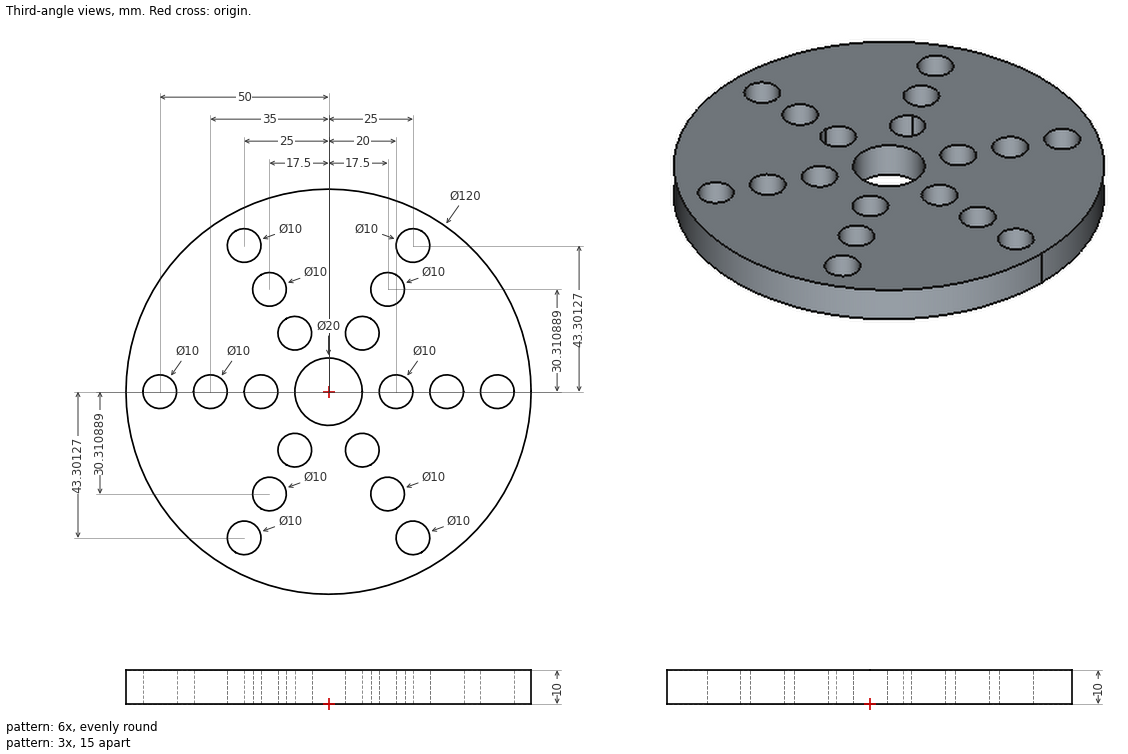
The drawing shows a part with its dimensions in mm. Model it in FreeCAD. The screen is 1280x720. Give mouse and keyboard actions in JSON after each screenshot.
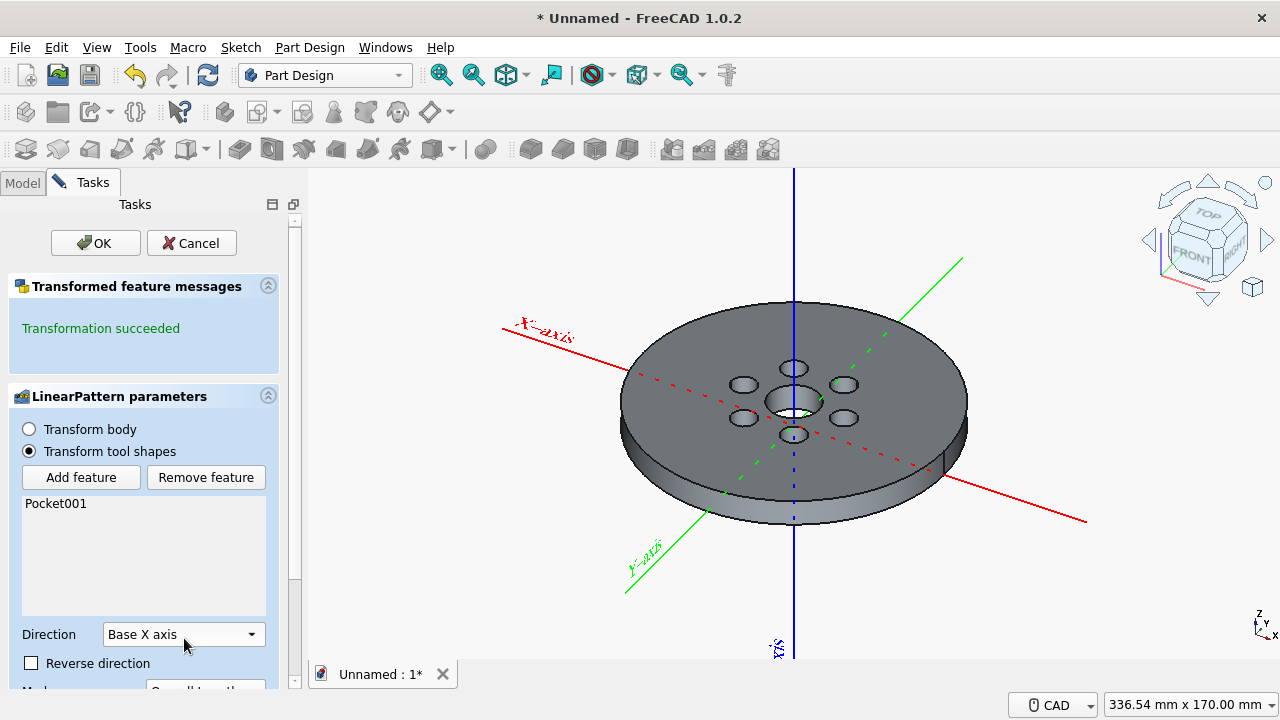
{"action": "scroll", "coordinate": [295, 451], "scroll_direction": "down", "scroll_amount": 2}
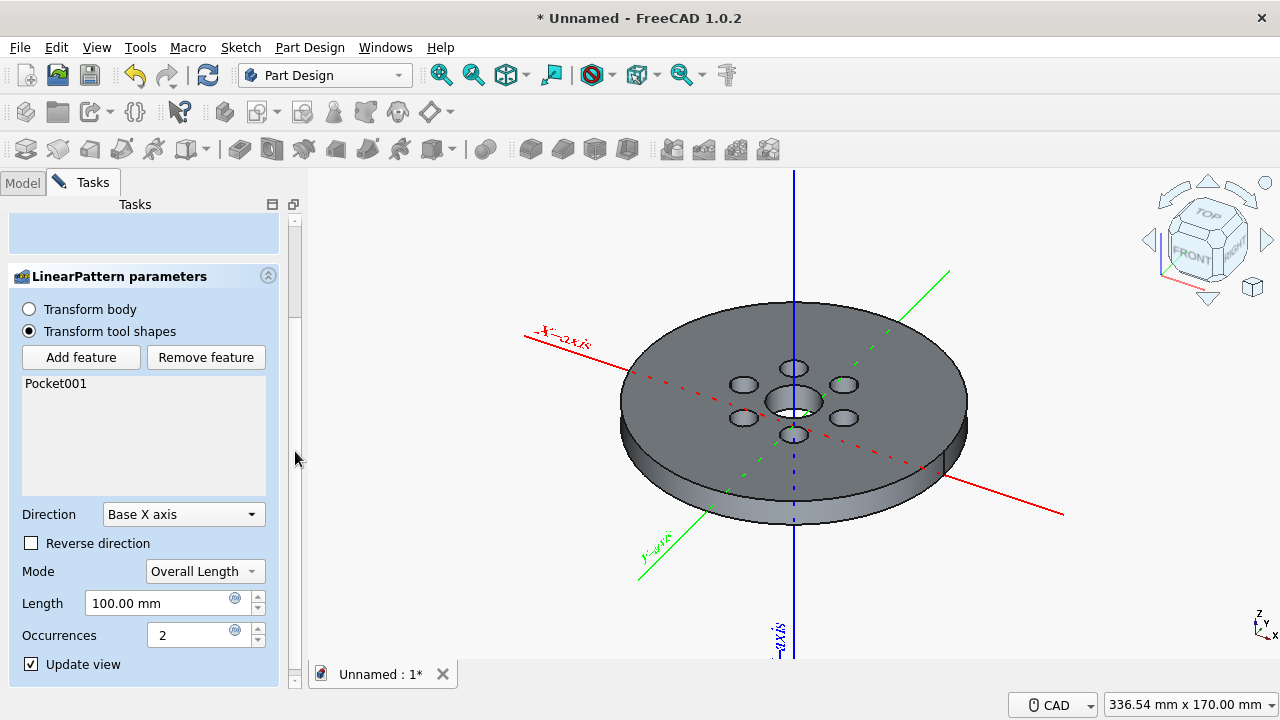
{"action": "left_click", "coordinate": [206, 572]}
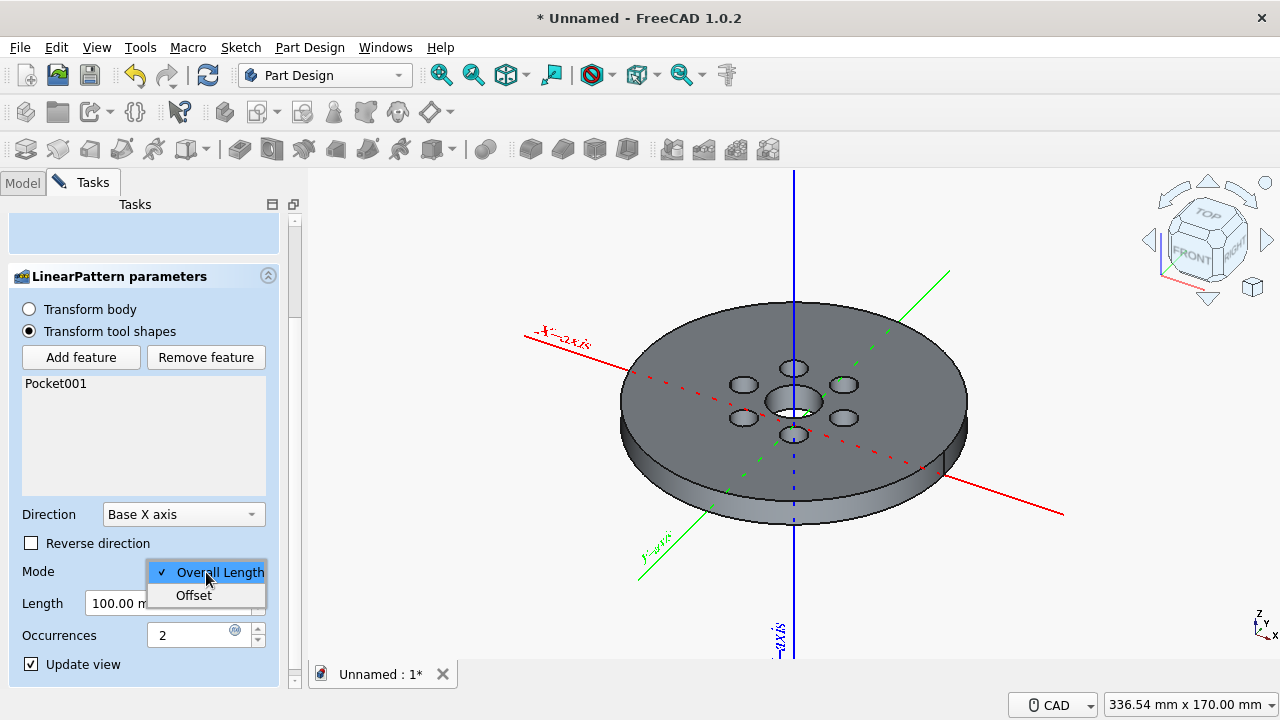
{"action": "left_click", "coordinate": [206, 596]}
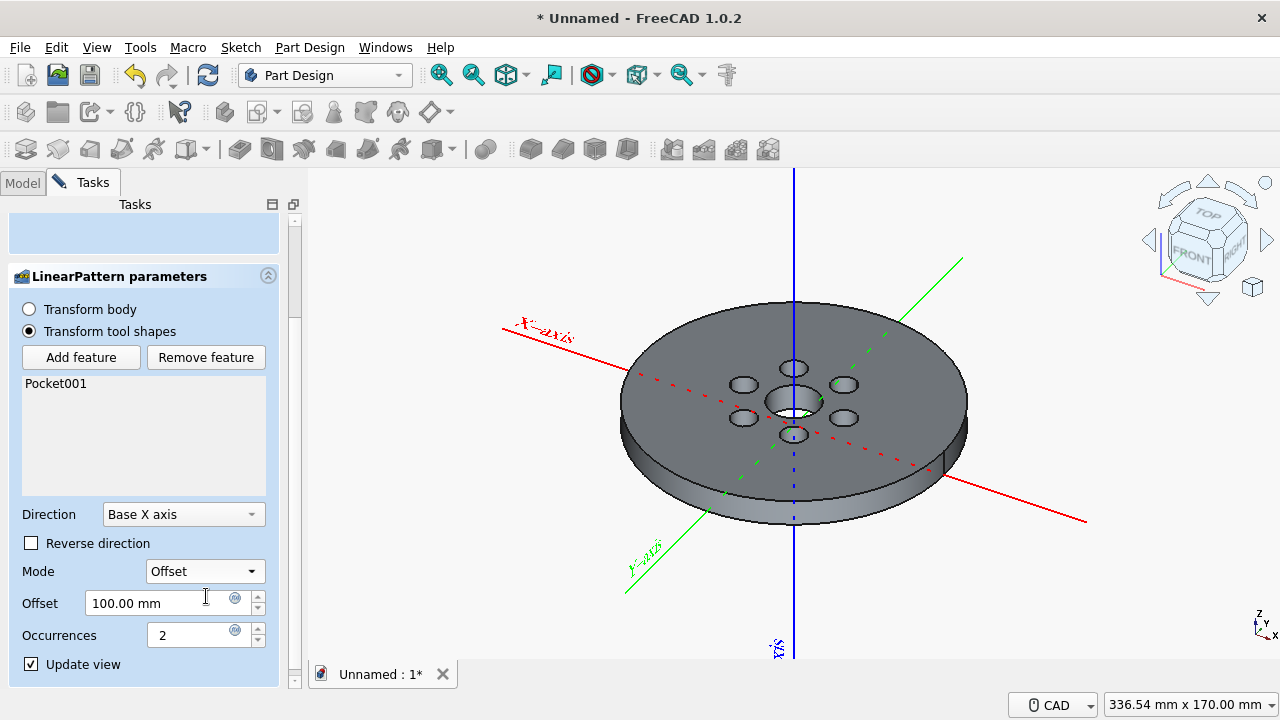
{"action": "triple_click", "coordinate": [168, 603]}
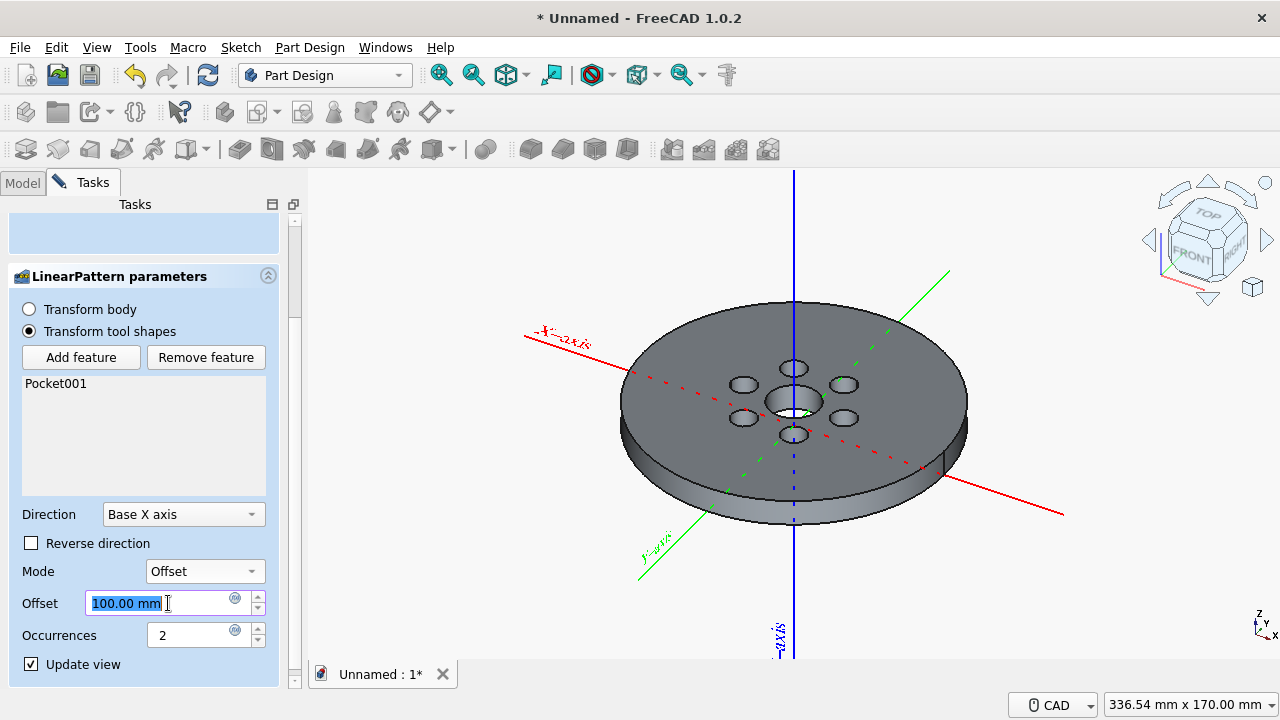
{"action": "type", "text": "15"}
{"action": "key", "text": "Tab"}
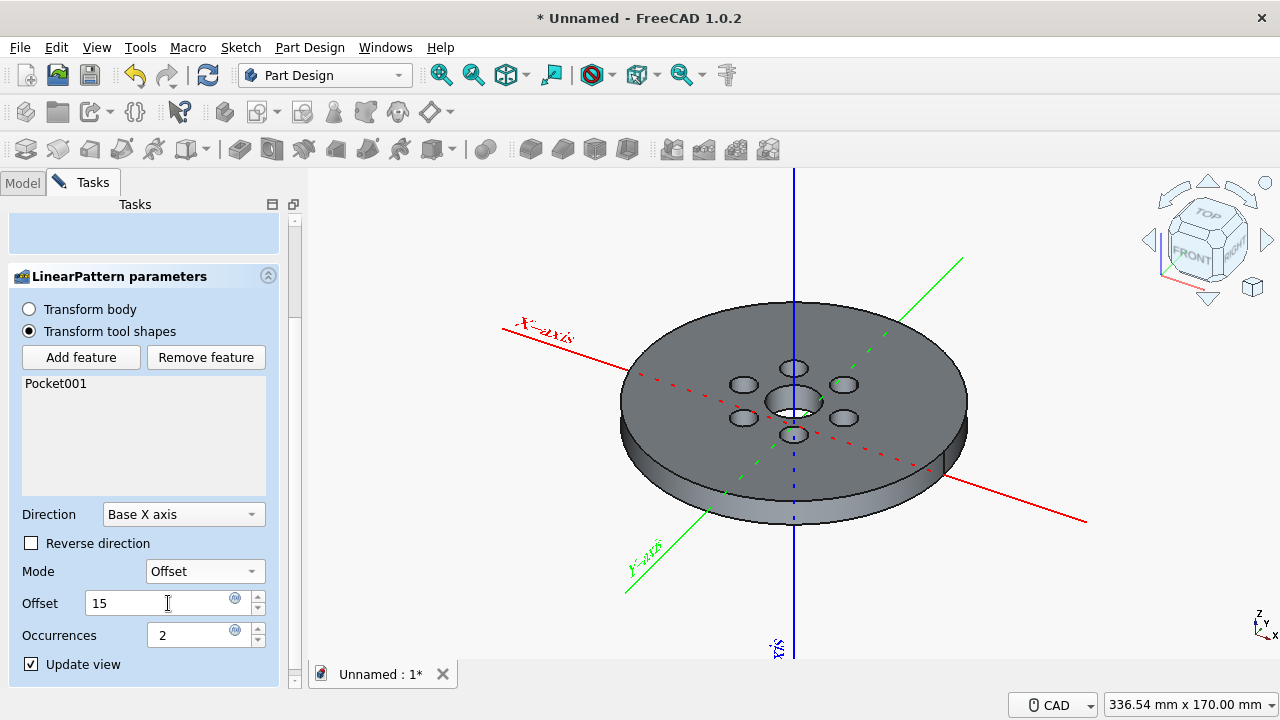
{"action": "triple_click", "coordinate": [198, 635]}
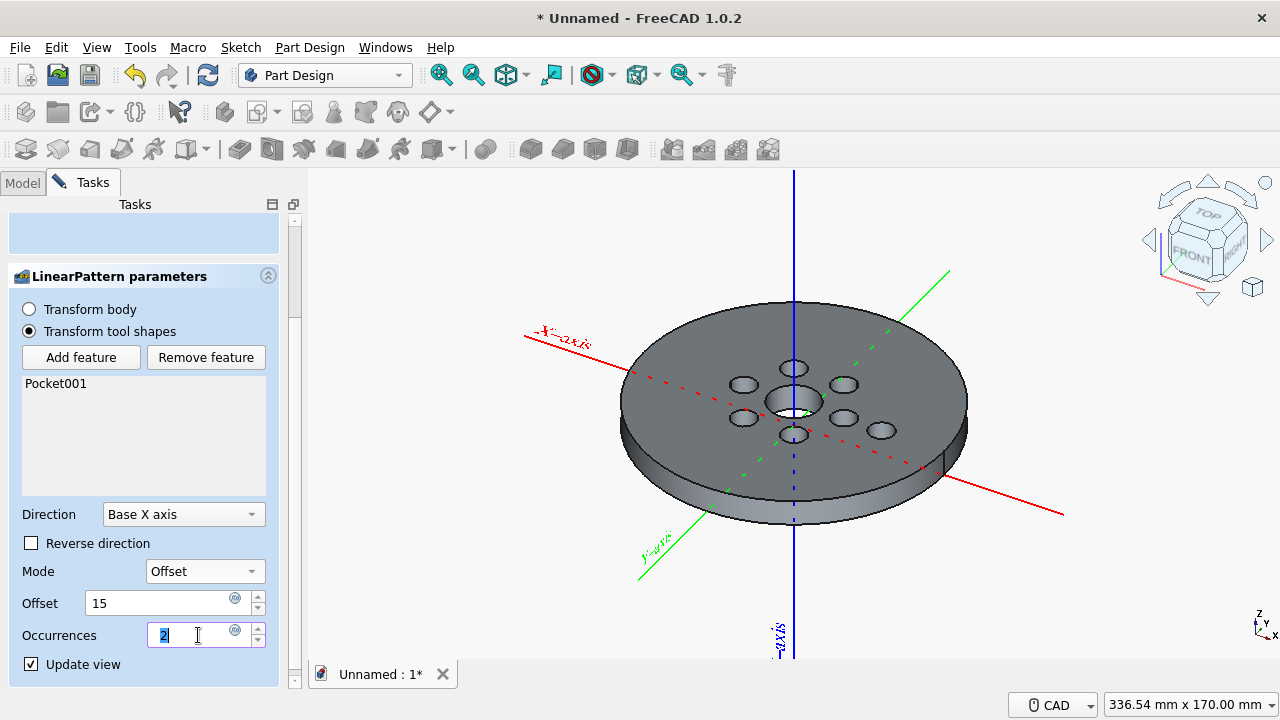
{"action": "type", "text": "3"}
{"action": "key", "text": "Tab"}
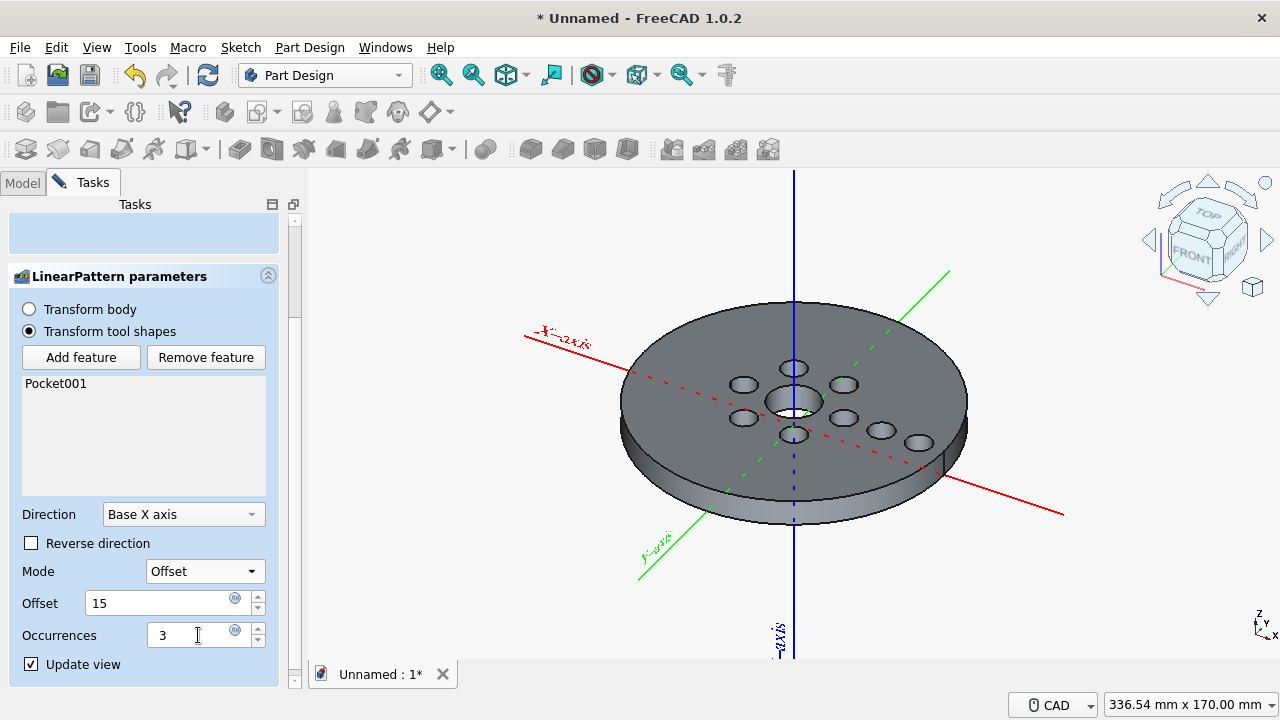
{"action": "scroll", "coordinate": [295, 451], "scroll_direction": "up", "scroll_amount": 3}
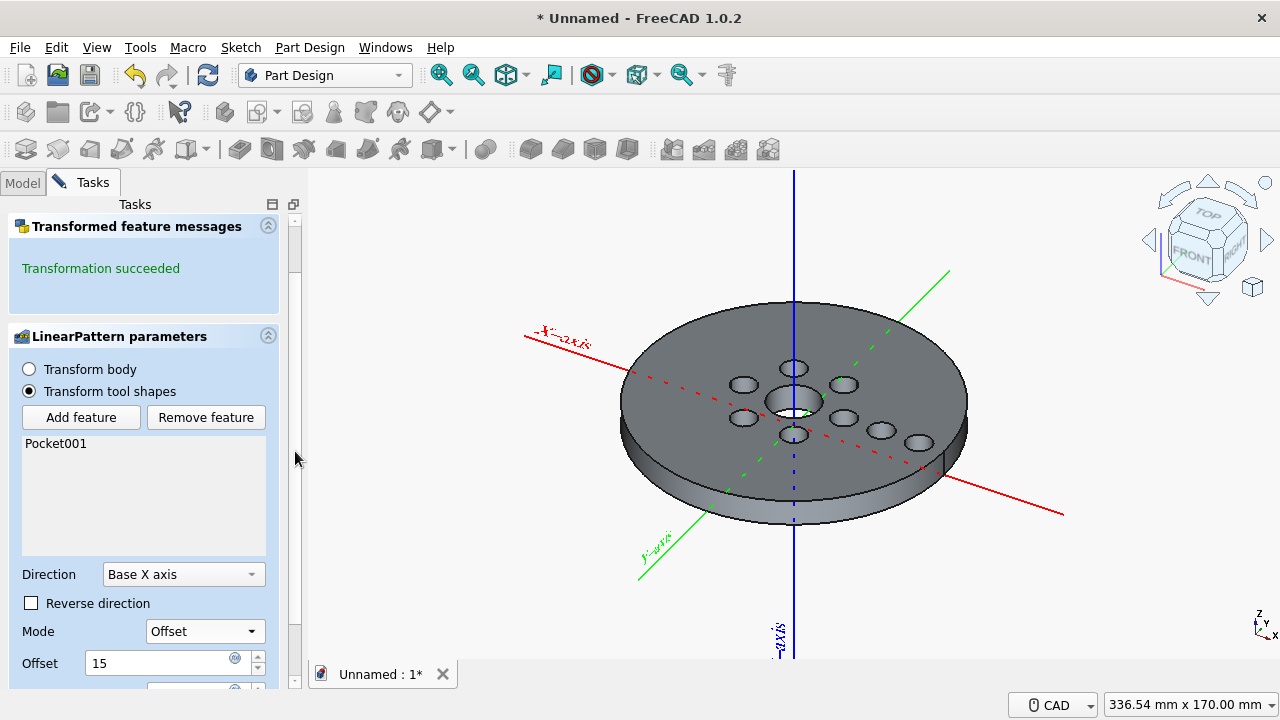
{"action": "left_click", "coordinate": [96, 243]}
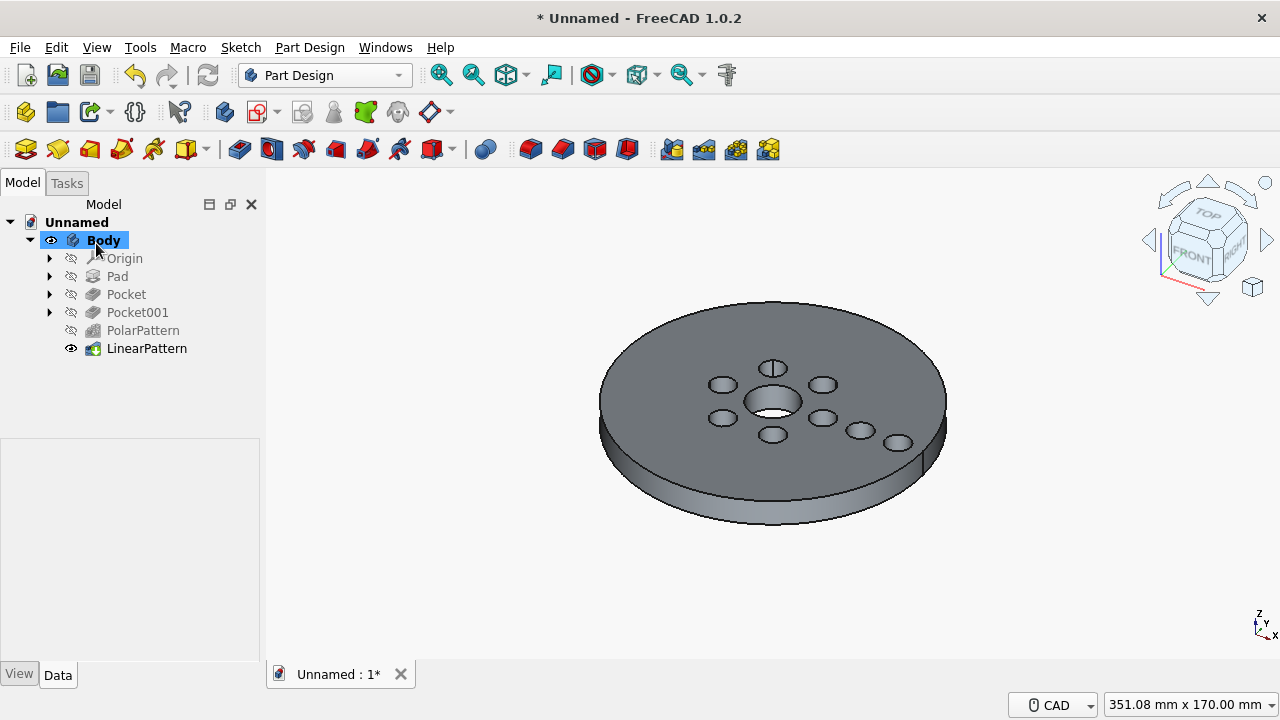
{"action": "left_click", "coordinate": [662, 397]}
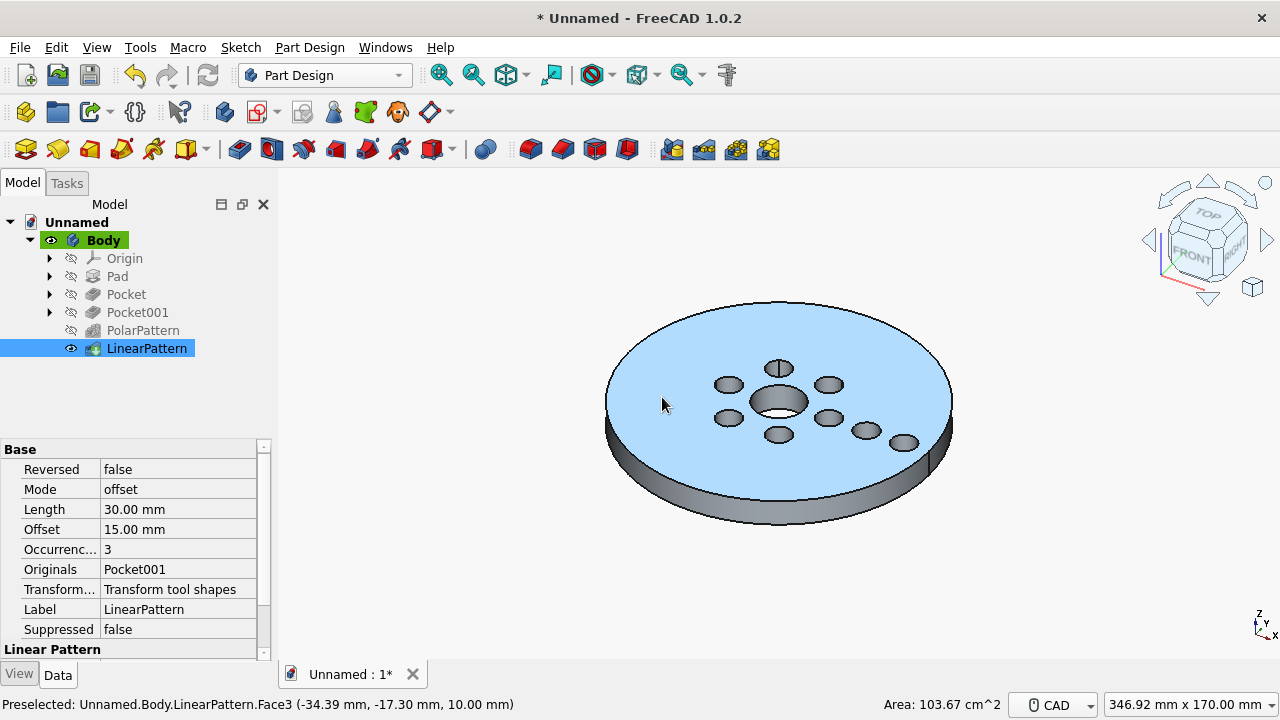
{"action": "left_click", "coordinate": [258, 112]}